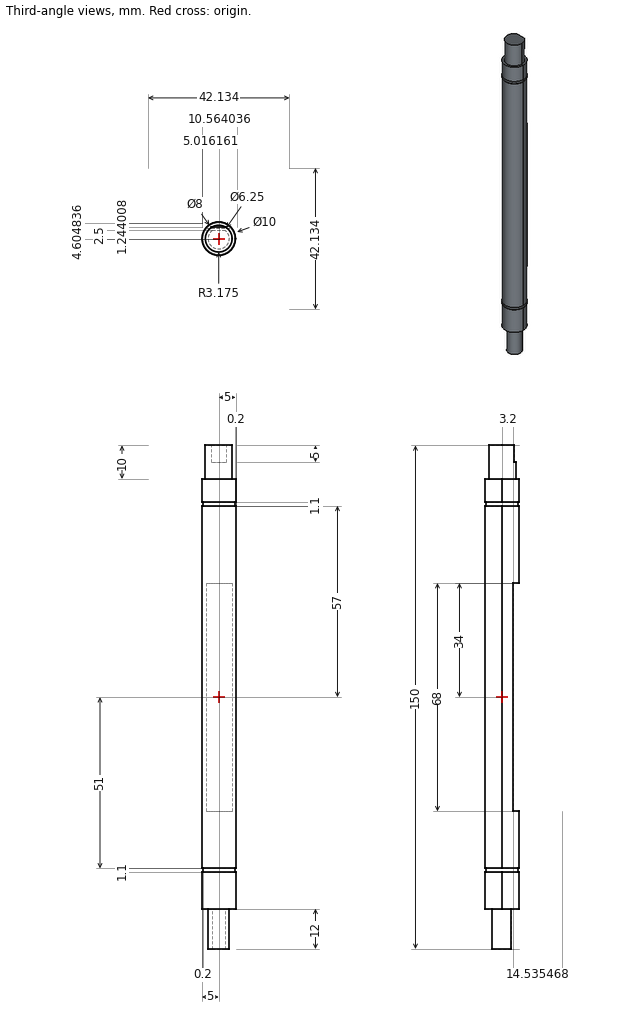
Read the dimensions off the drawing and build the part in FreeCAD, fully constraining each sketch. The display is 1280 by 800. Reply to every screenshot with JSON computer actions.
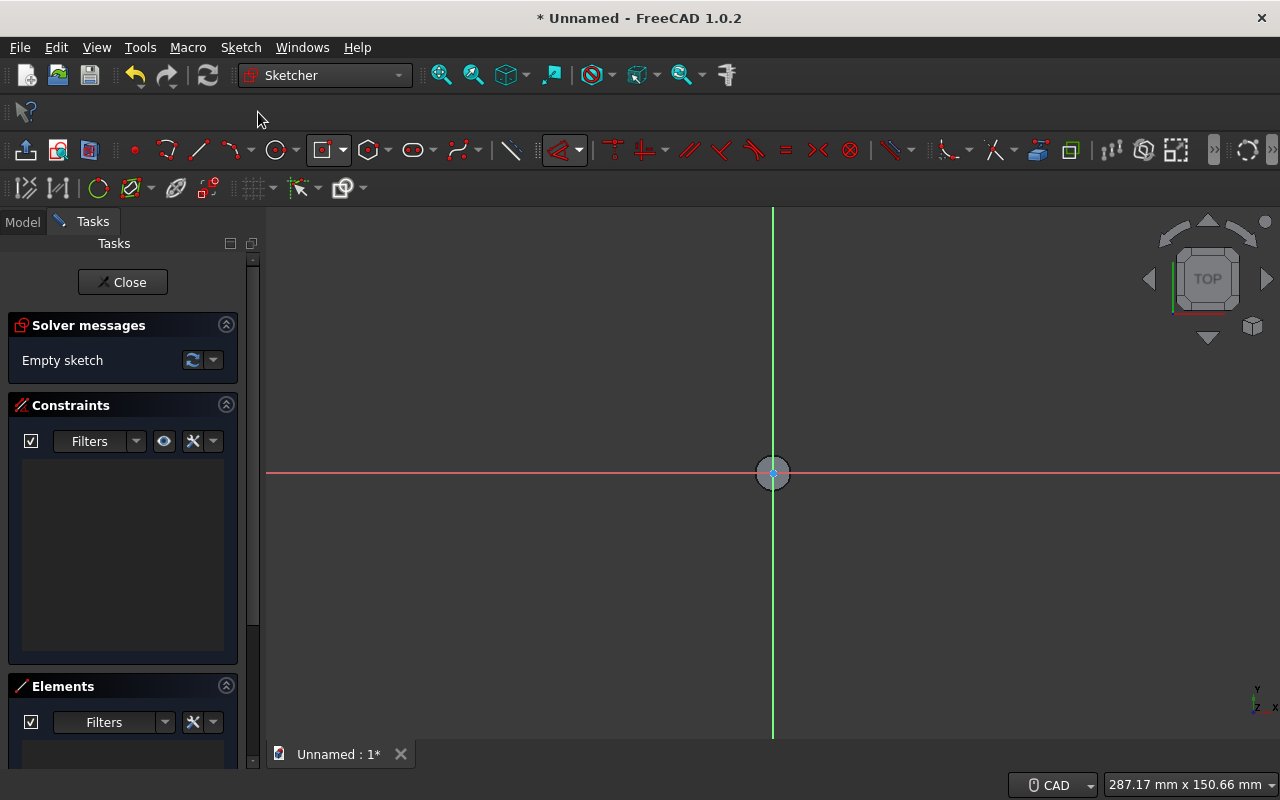
{"action": "scroll", "coordinate": [829, 473], "scroll_direction": "up", "scroll_amount": 4}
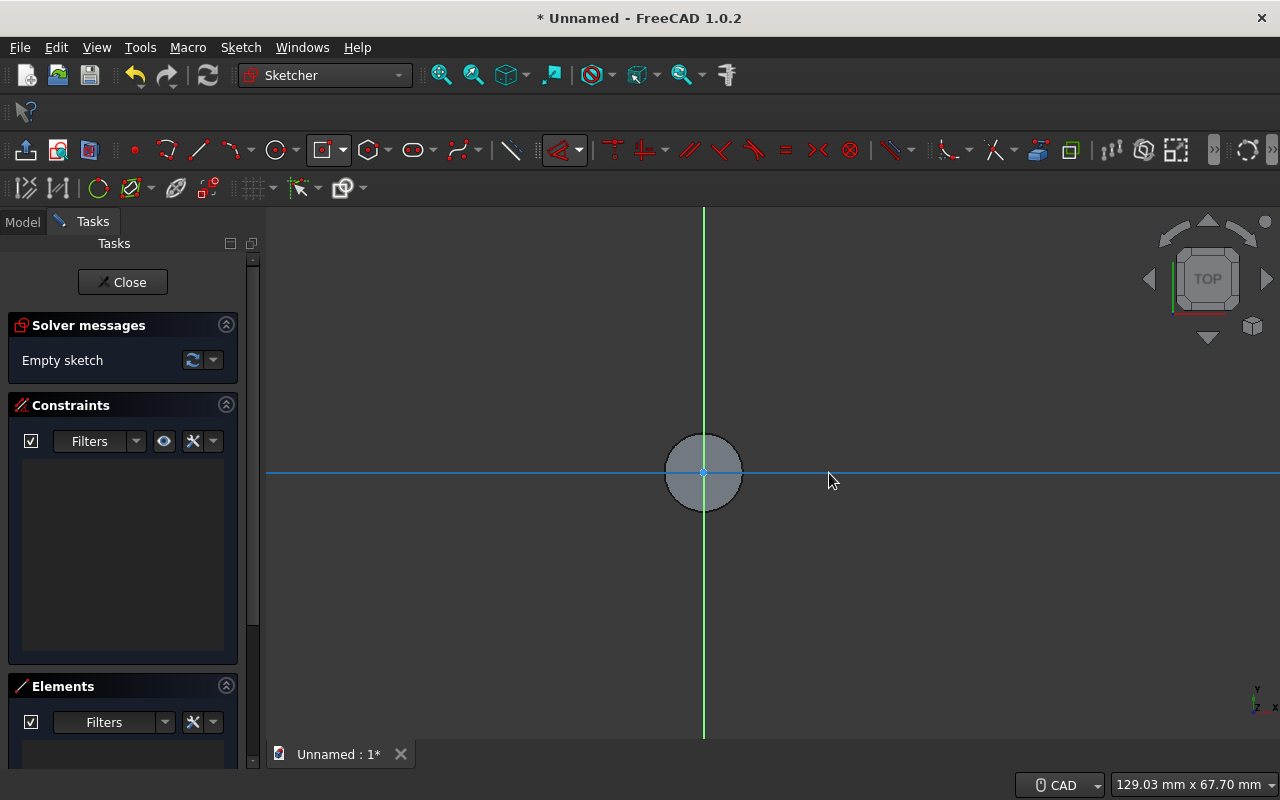
{"action": "left_click", "coordinate": [322, 150]}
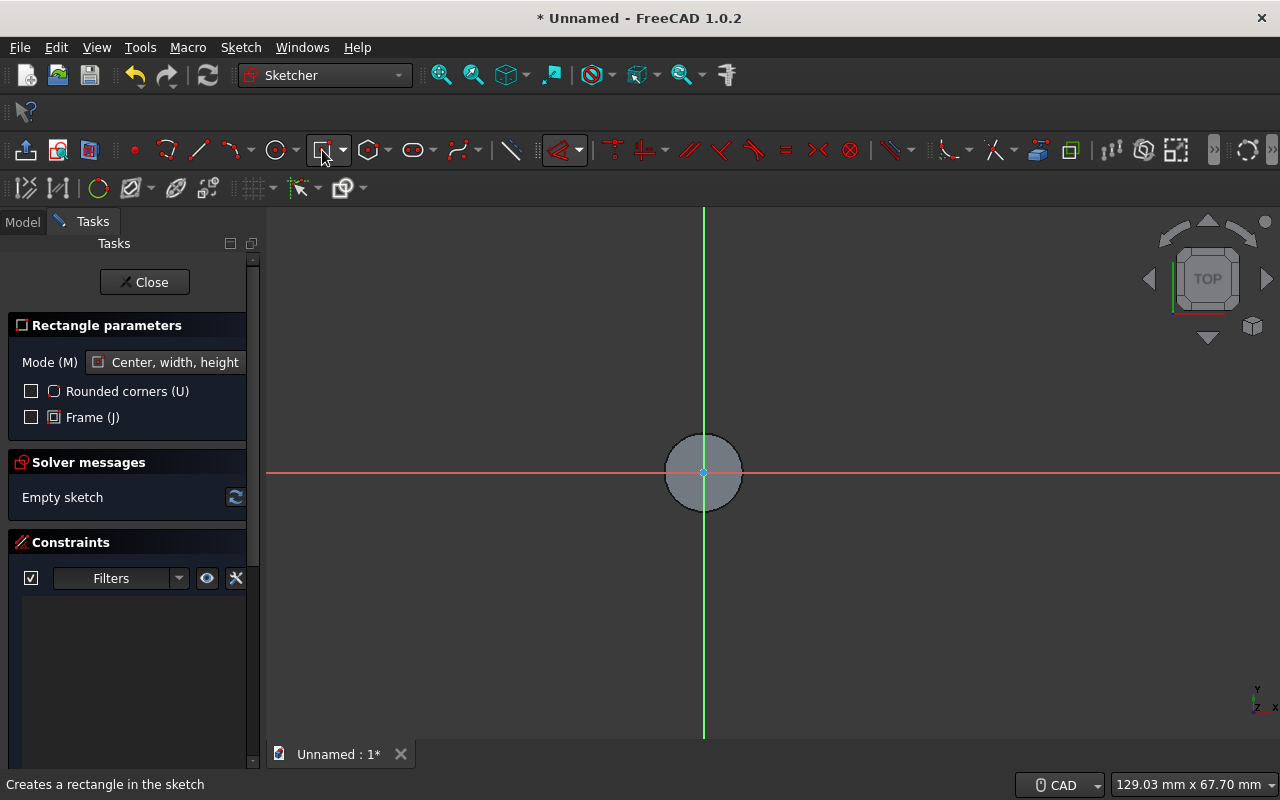
{"action": "left_click", "coordinate": [704, 473]}
{"action": "left_click", "coordinate": [869, 307]}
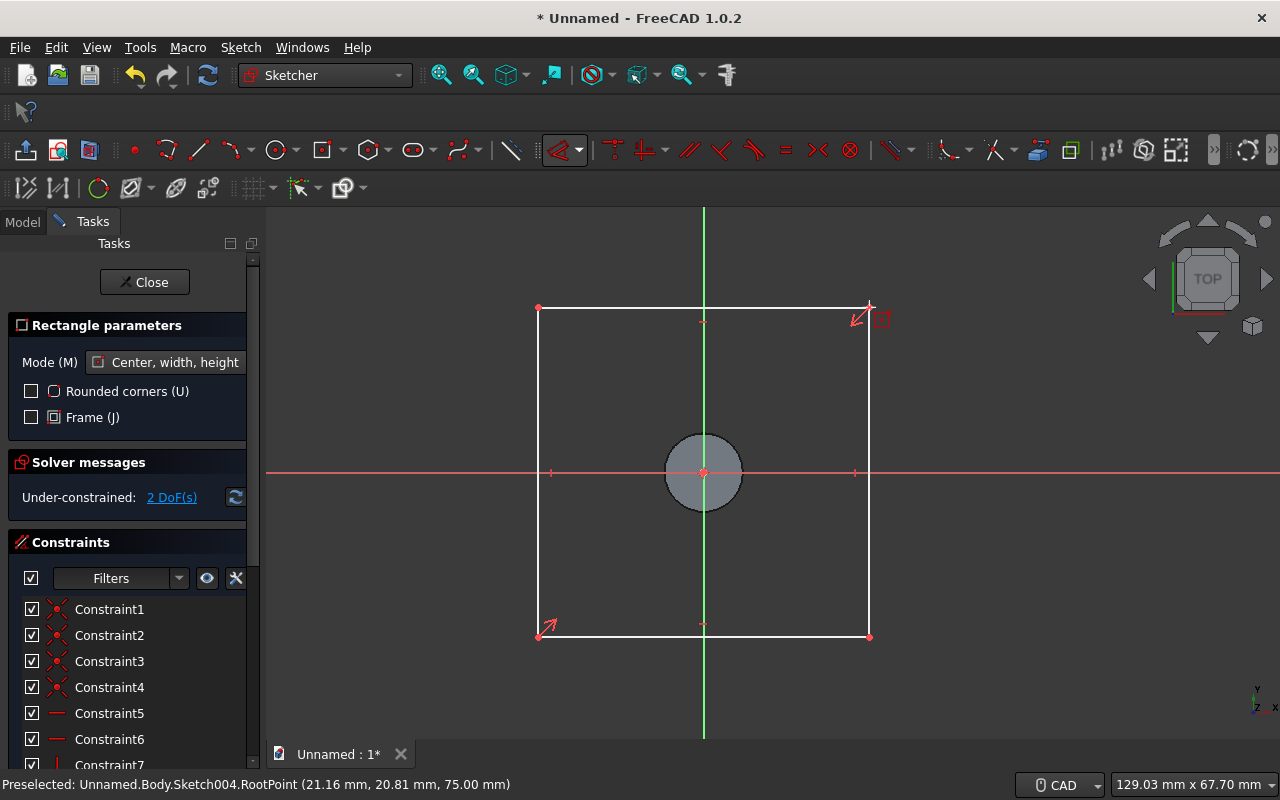
{"action": "left_click", "coordinate": [276, 150]}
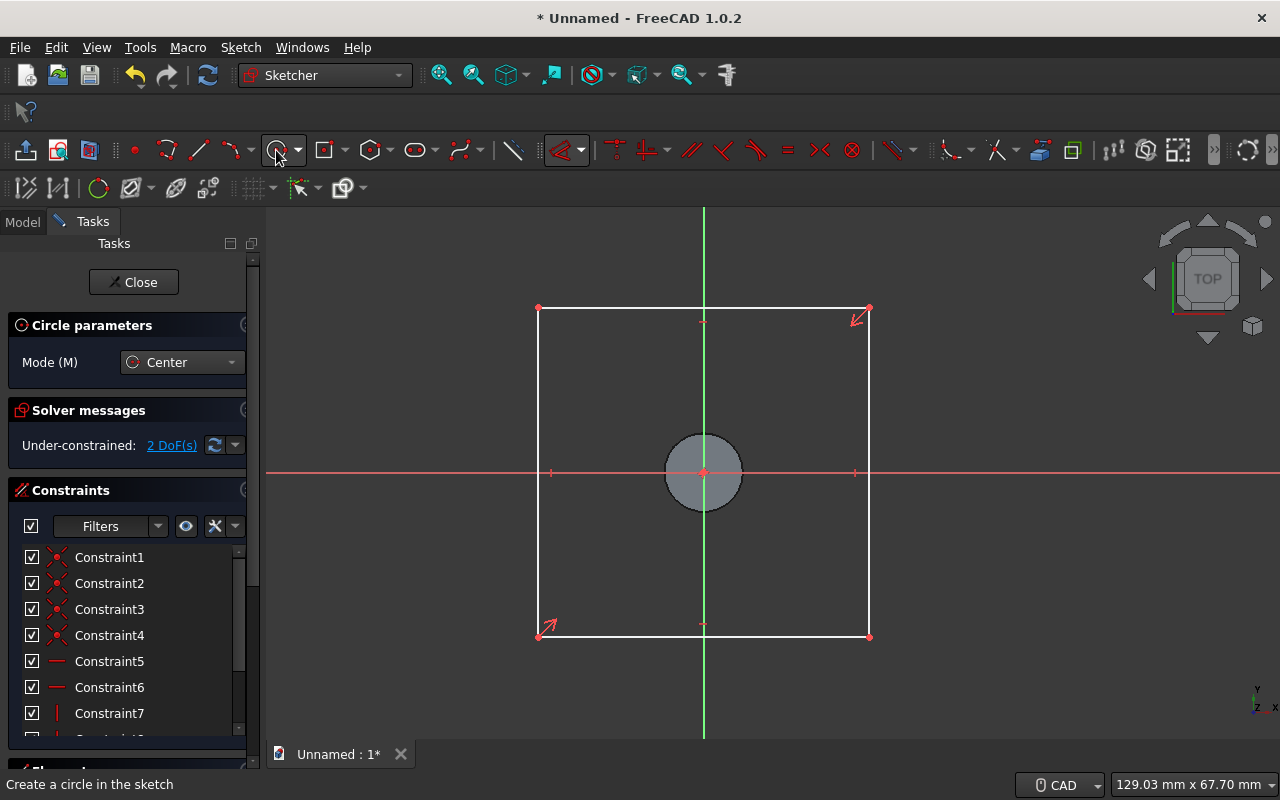
{"action": "left_click", "coordinate": [704, 473]}
{"action": "left_click", "coordinate": [726, 450]}
{"action": "key", "text": "Escape"}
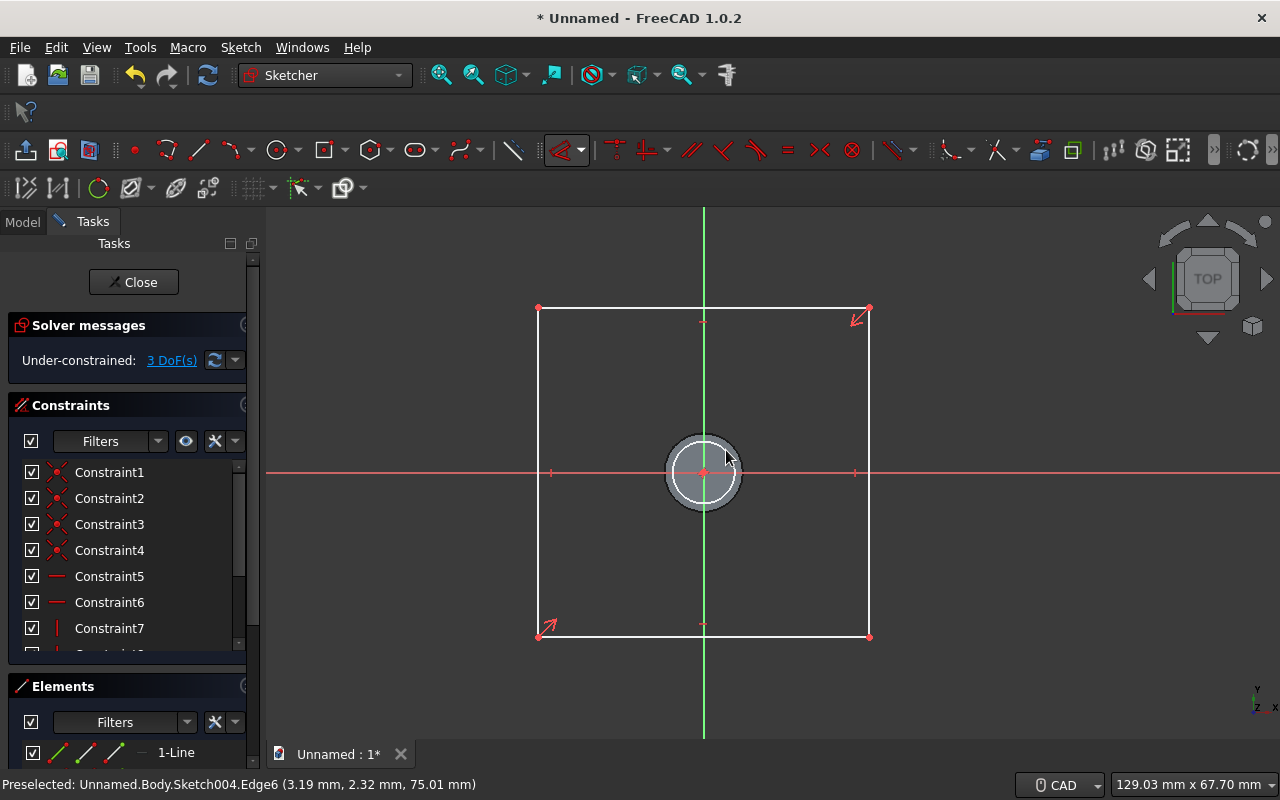
{"action": "left_click", "coordinate": [726, 451]}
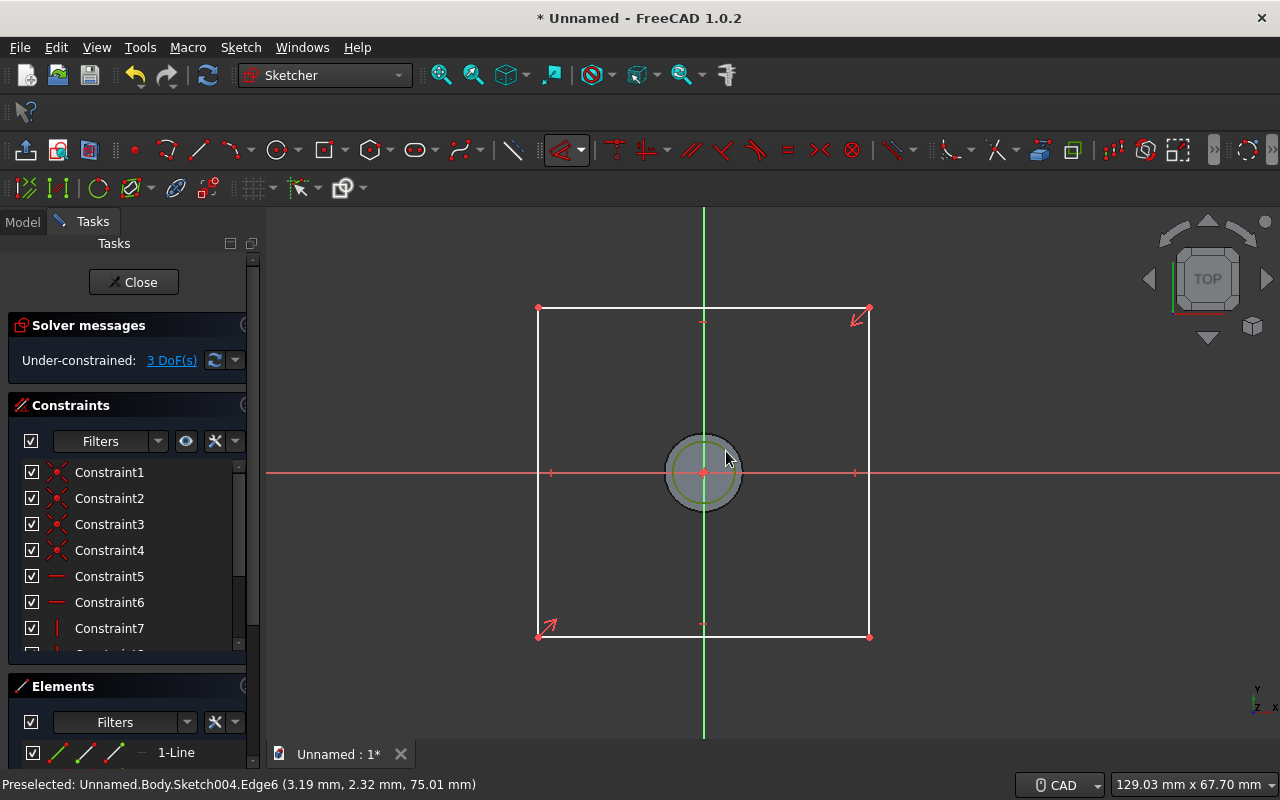
{"action": "left_click", "coordinate": [584, 150]}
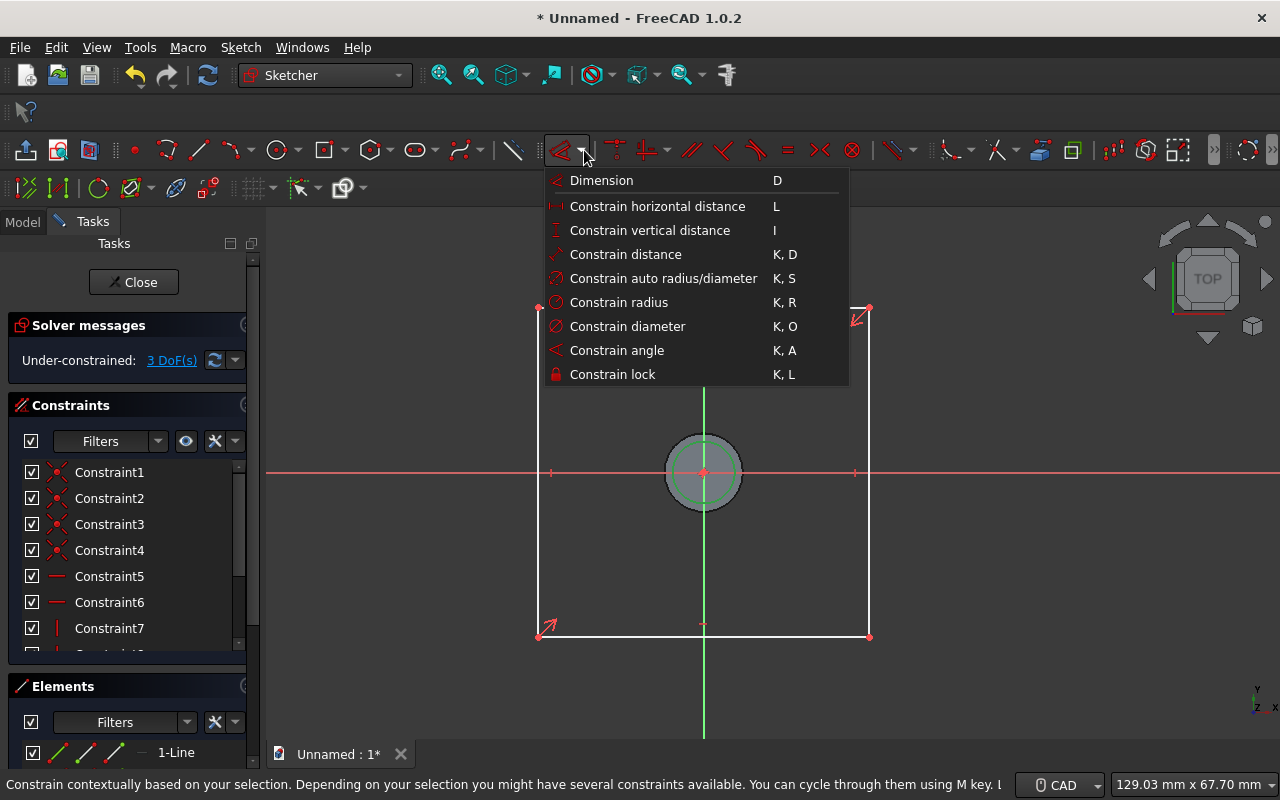
{"action": "left_click", "coordinate": [697, 326]}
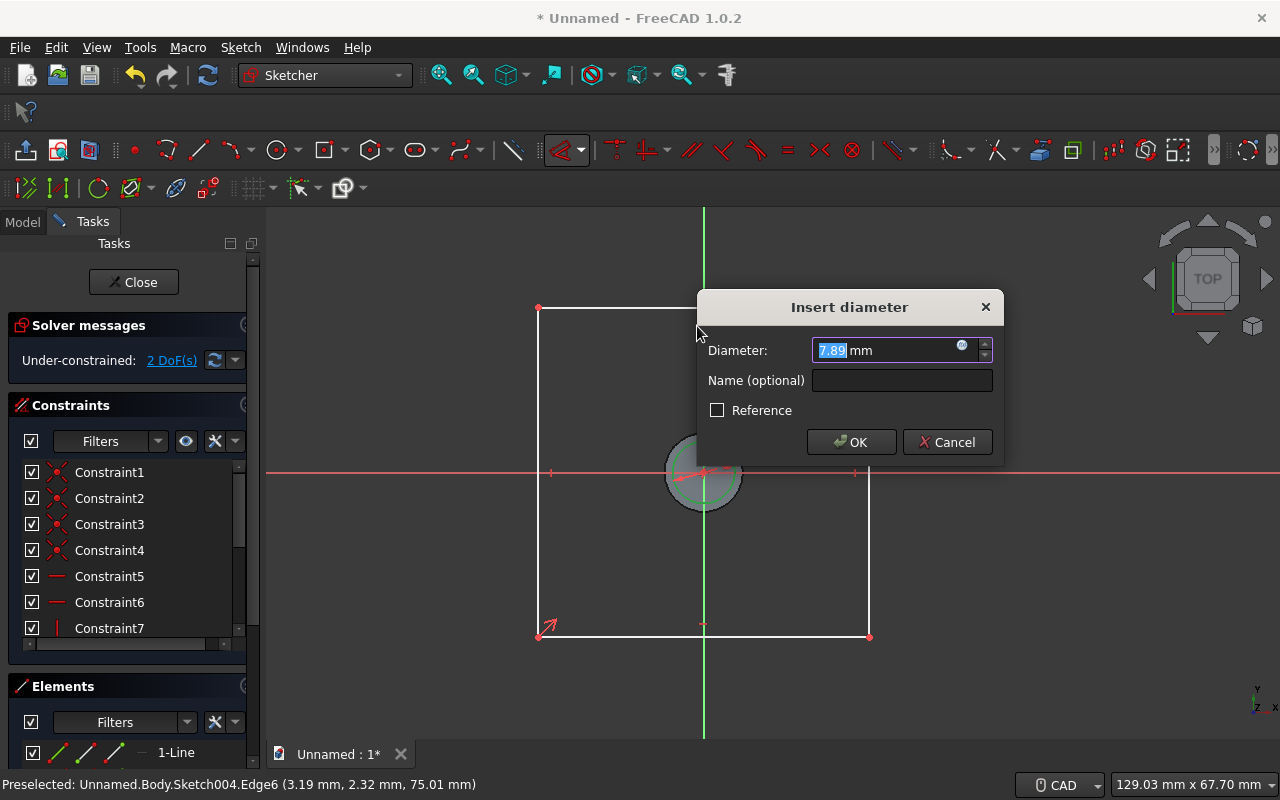
{"action": "type", "text": "8"}
{"action": "key", "text": "Return"}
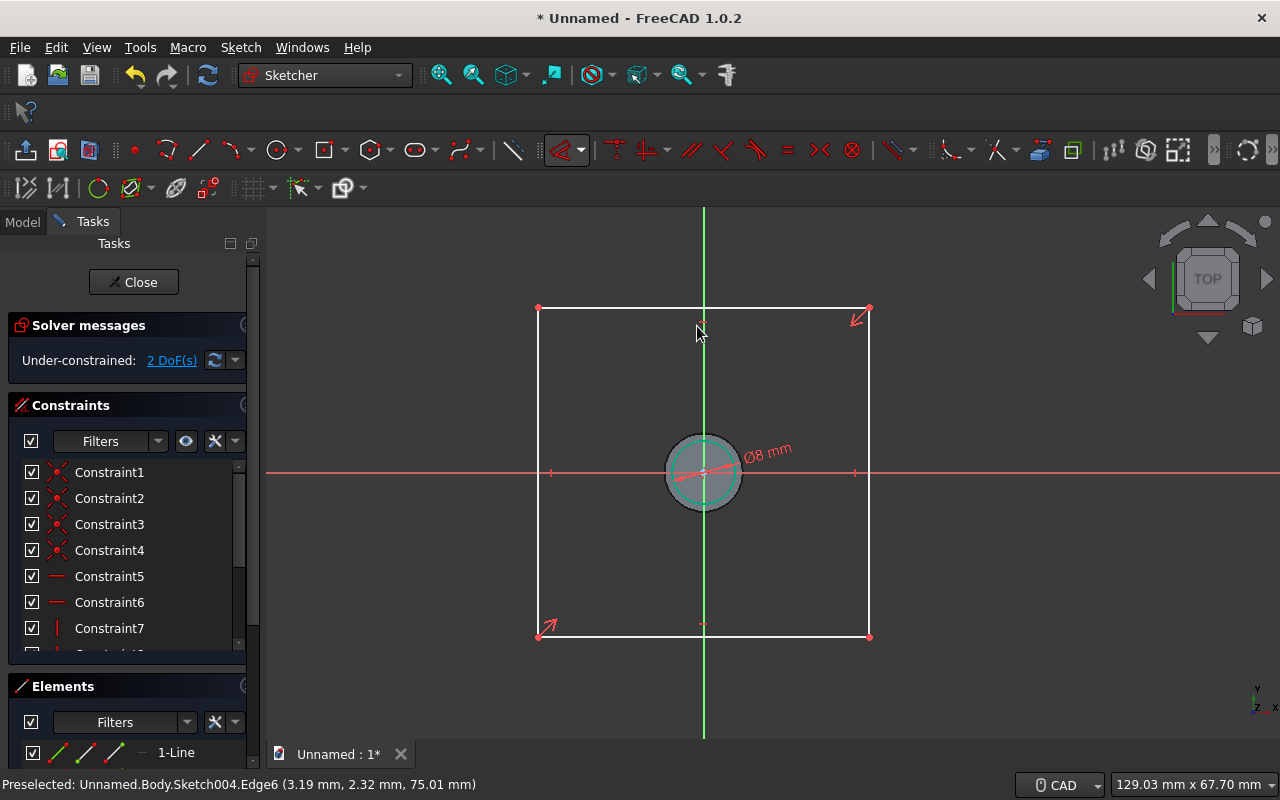
{"action": "left_click", "coordinate": [638, 637]}